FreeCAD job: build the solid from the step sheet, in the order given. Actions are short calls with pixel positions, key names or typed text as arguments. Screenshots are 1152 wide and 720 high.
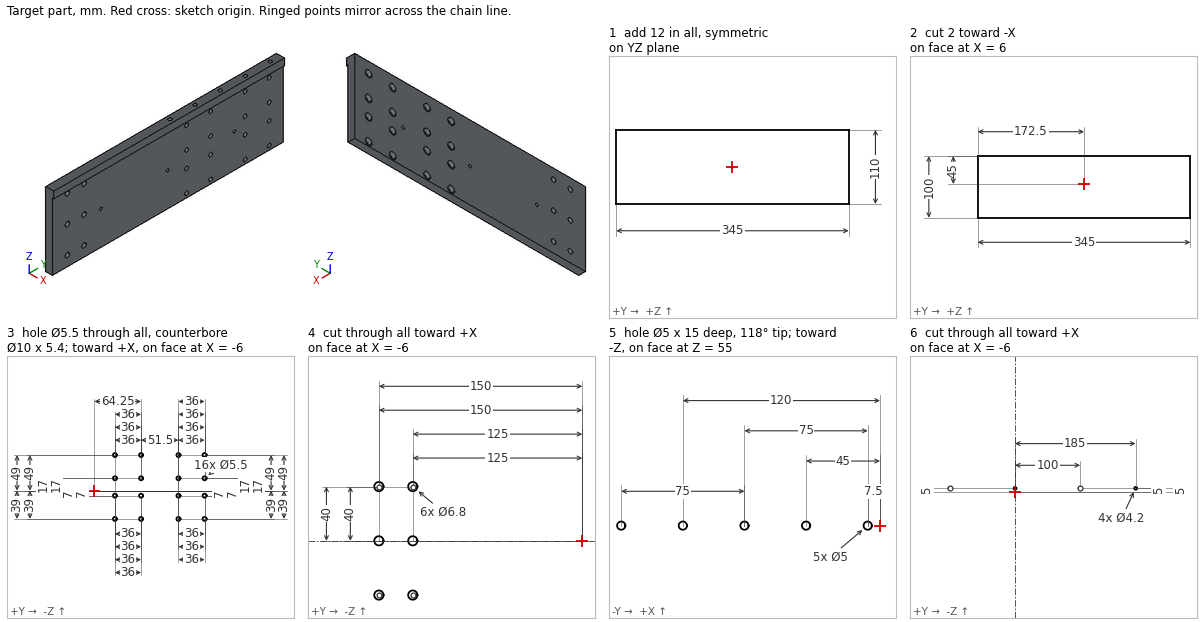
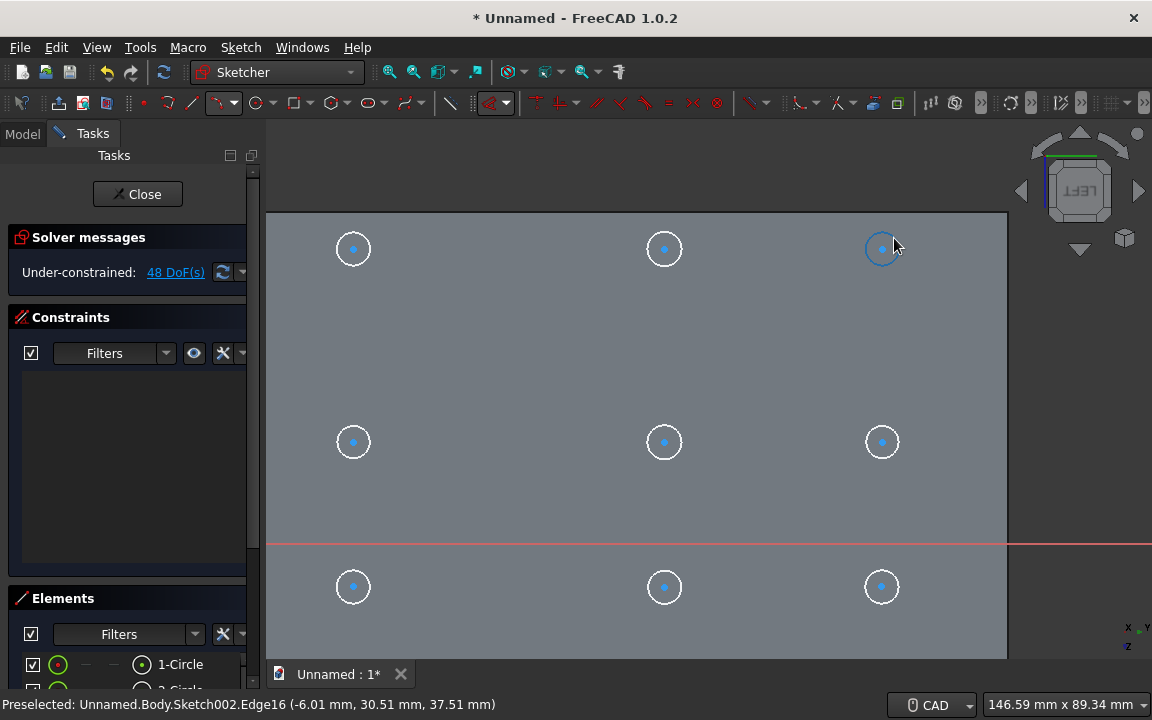
click(894, 237)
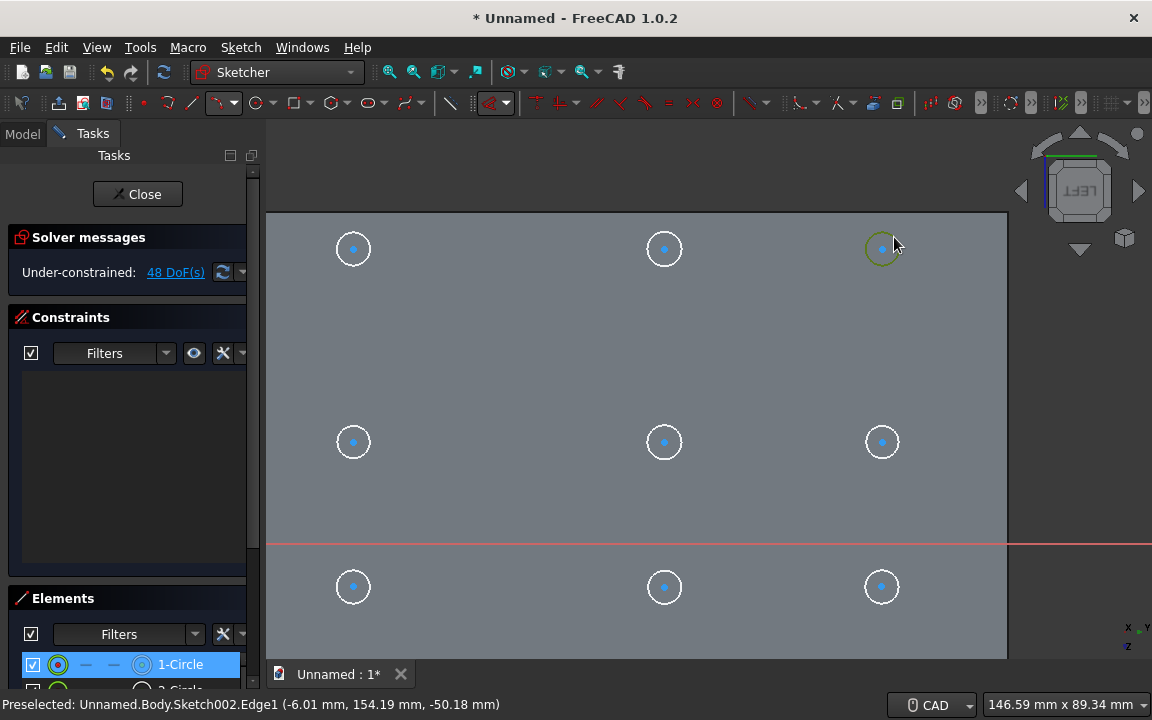
click(894, 431)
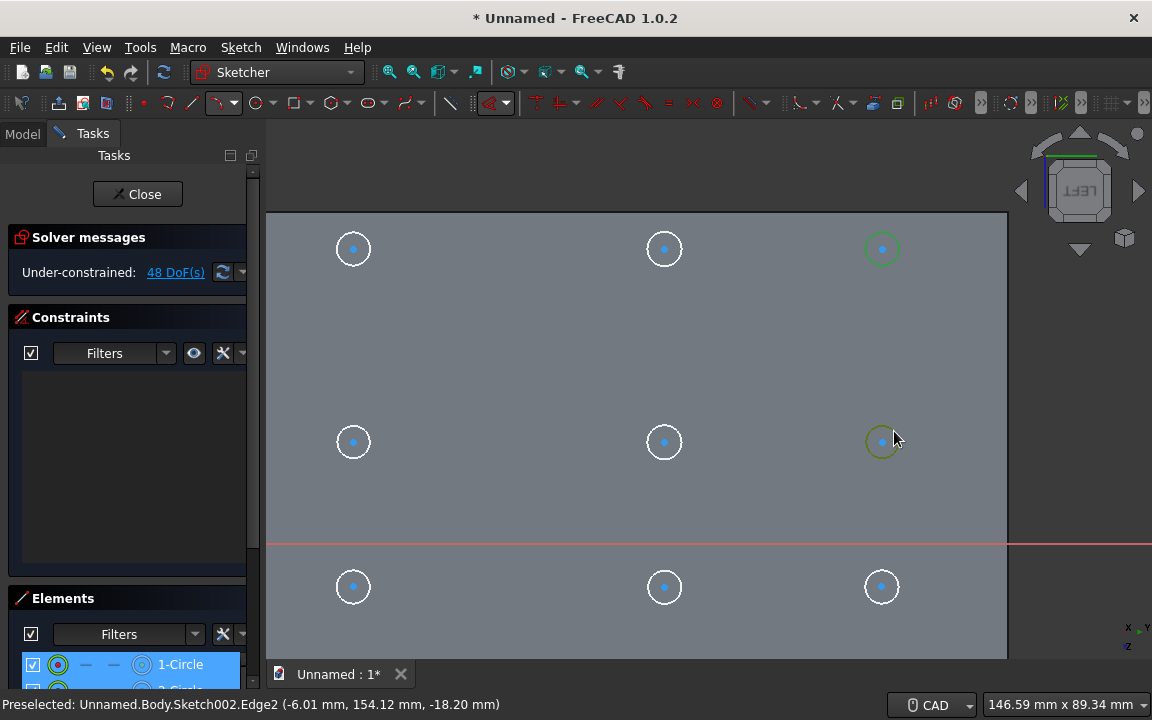
click(894, 575)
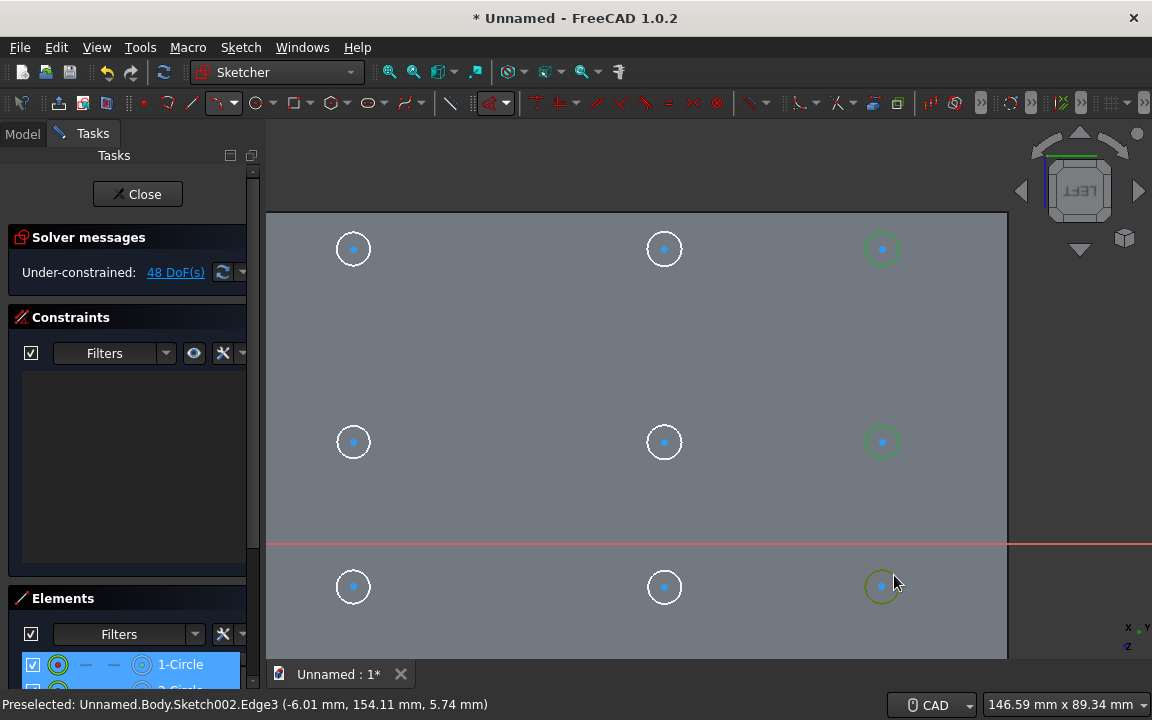
scroll(894, 237, down, 3)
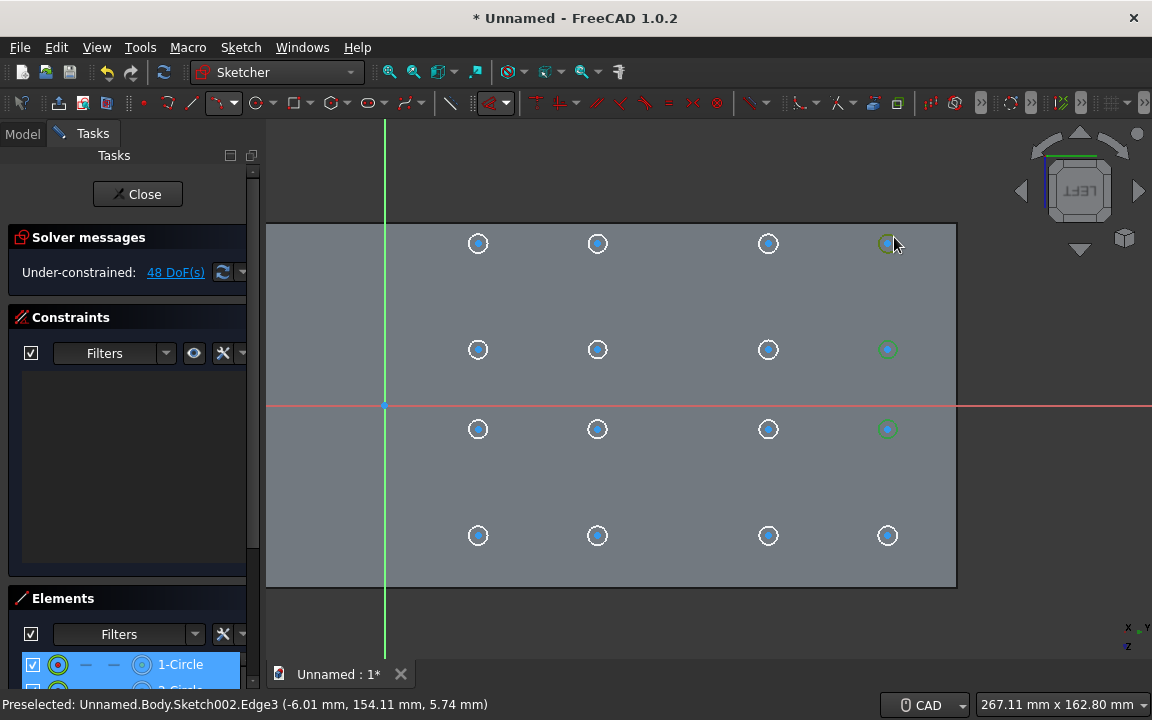
scroll(894, 529, up, 2)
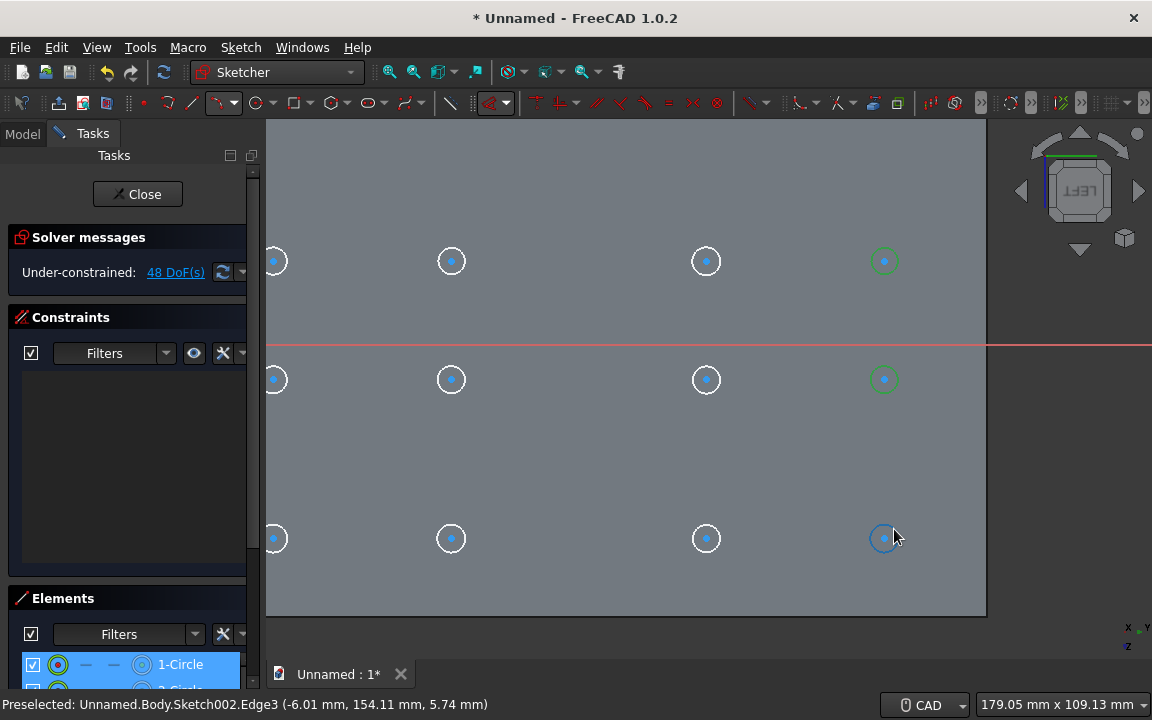
click(894, 529)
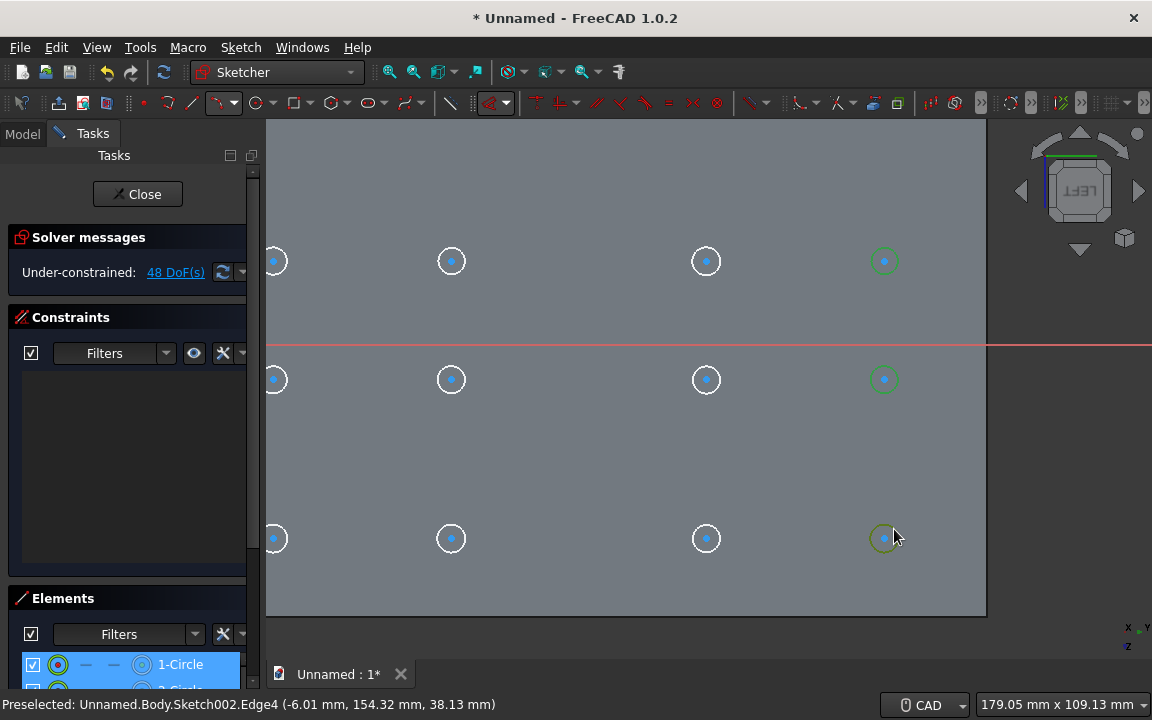
click(716, 529)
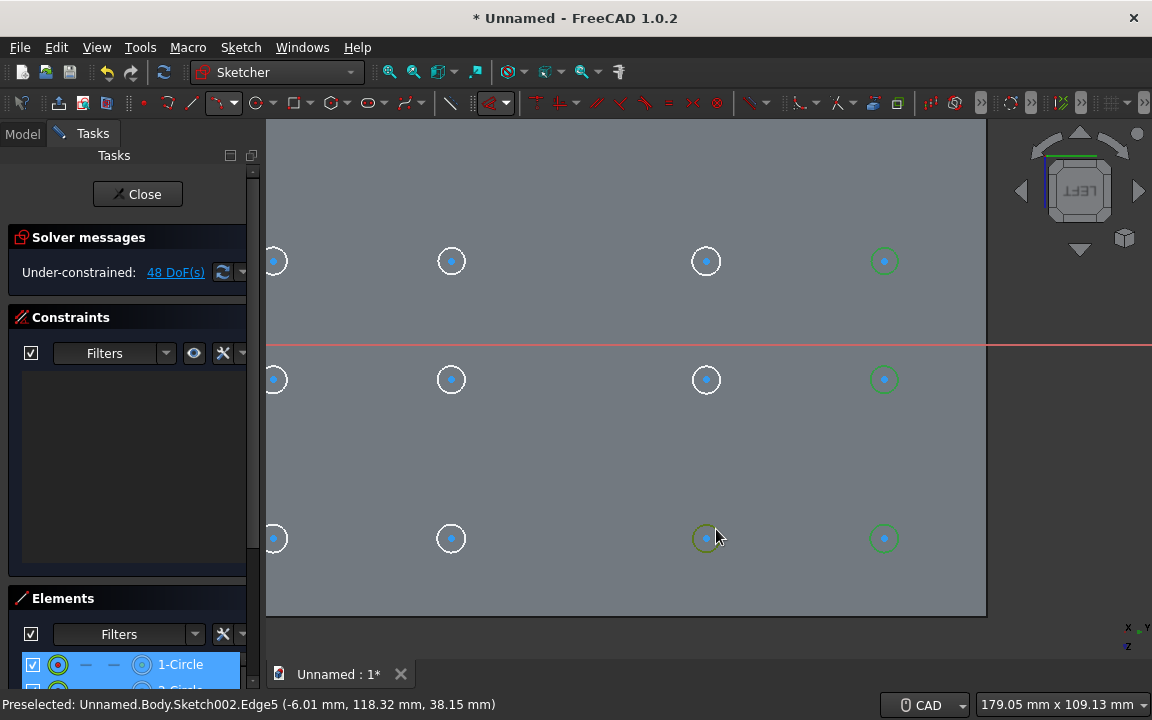
click(716, 370)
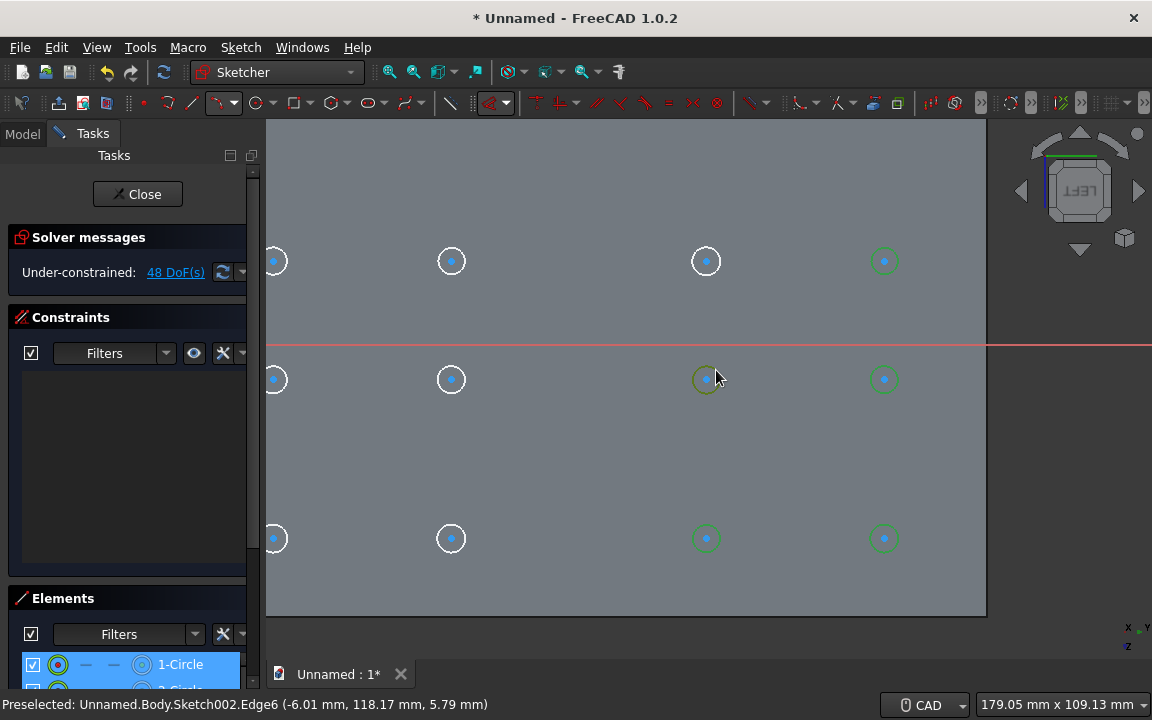
click(716, 251)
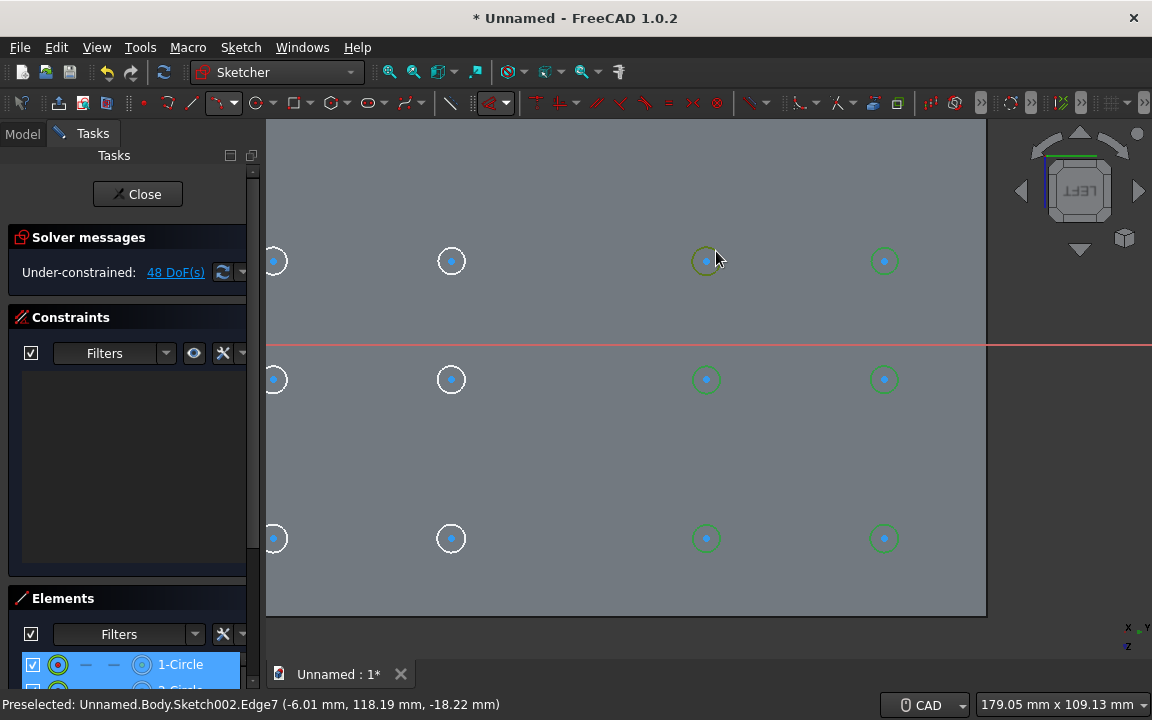
scroll(894, 529, down, 2)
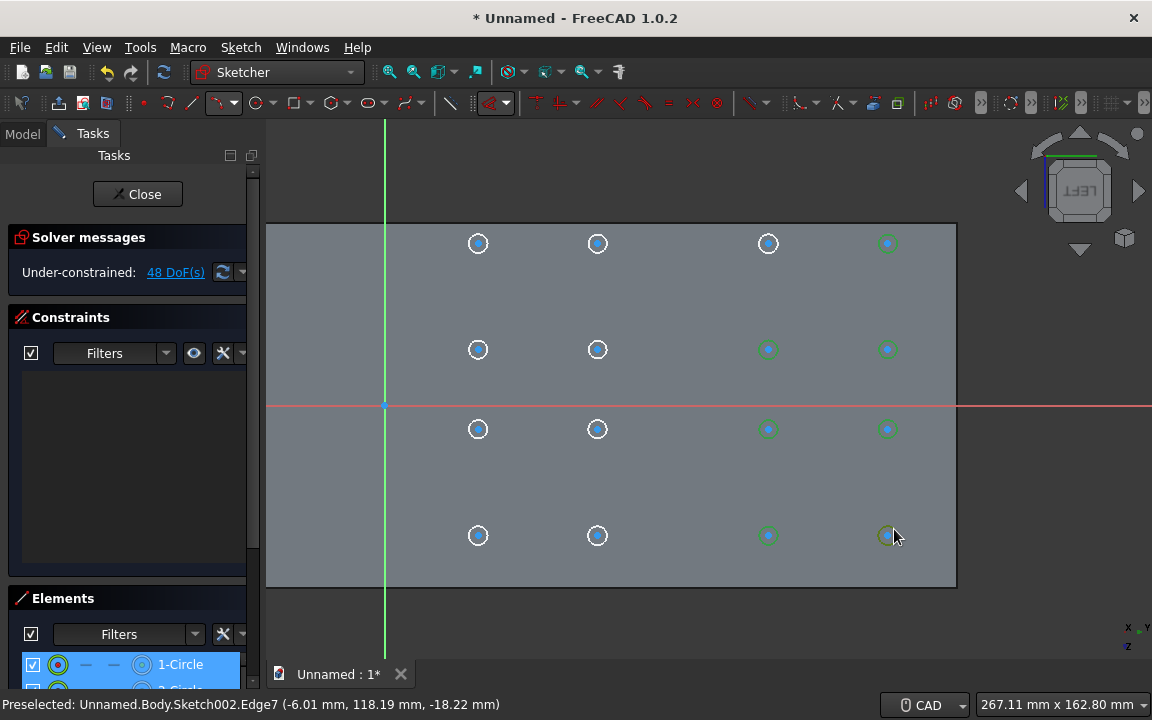
scroll(775, 237, up, 2)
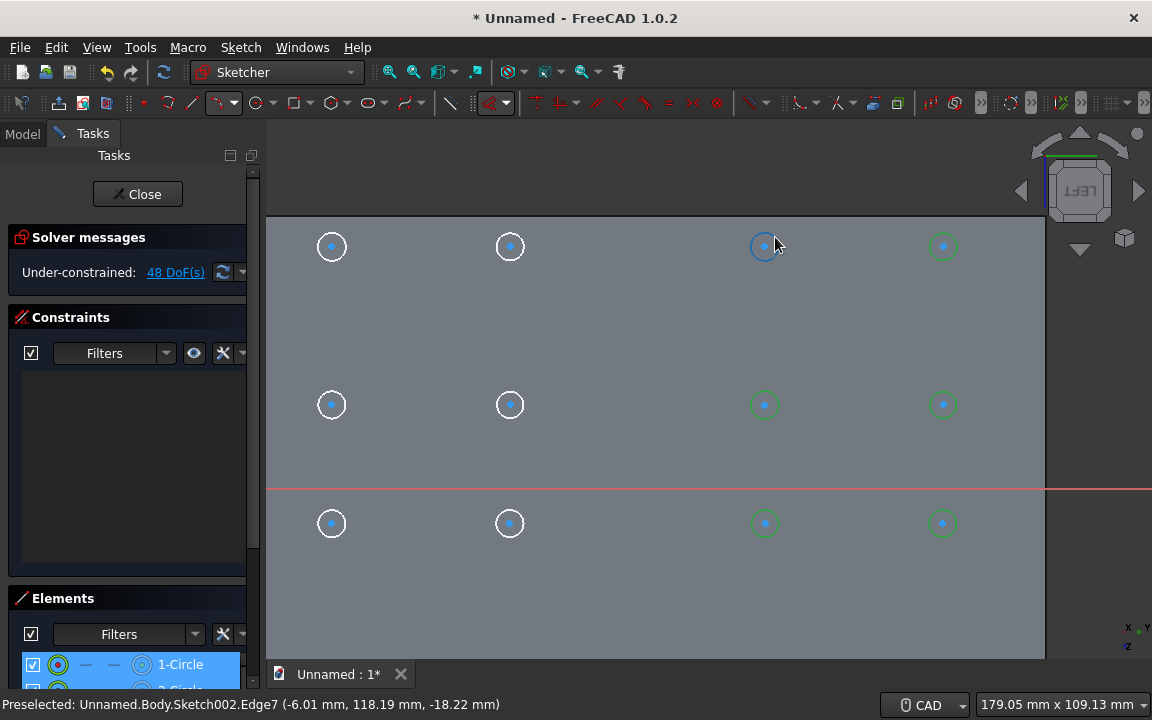
click(775, 237)